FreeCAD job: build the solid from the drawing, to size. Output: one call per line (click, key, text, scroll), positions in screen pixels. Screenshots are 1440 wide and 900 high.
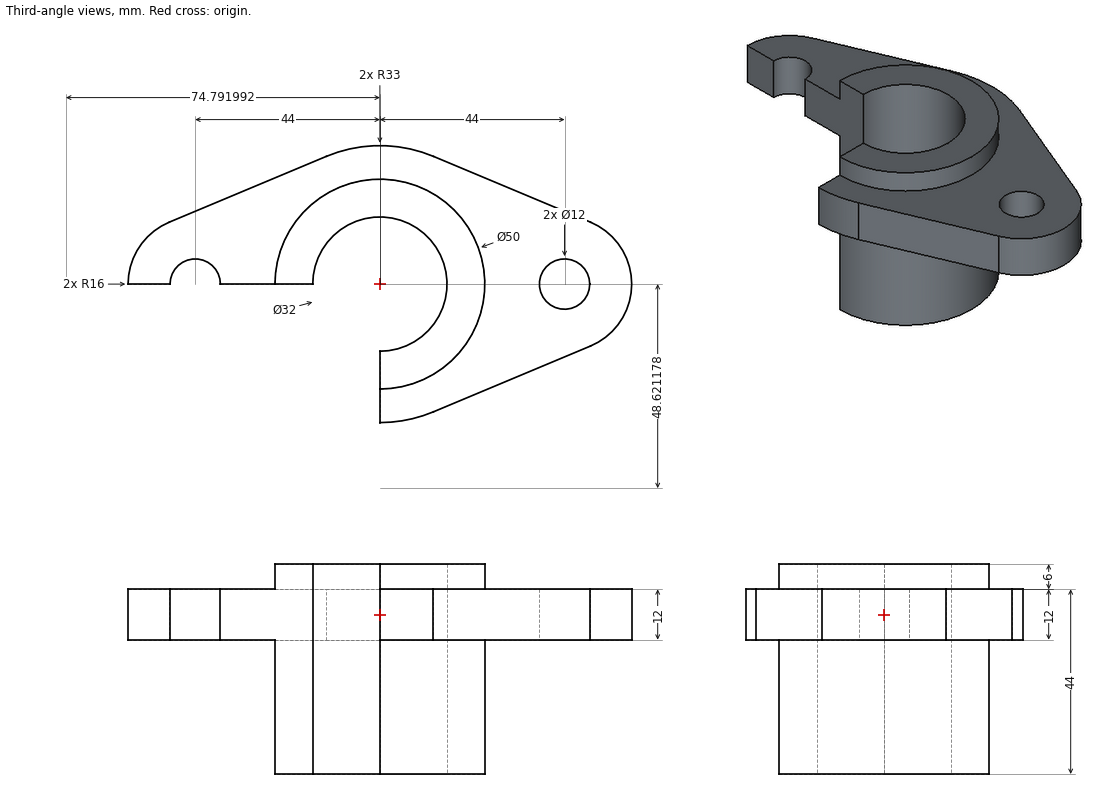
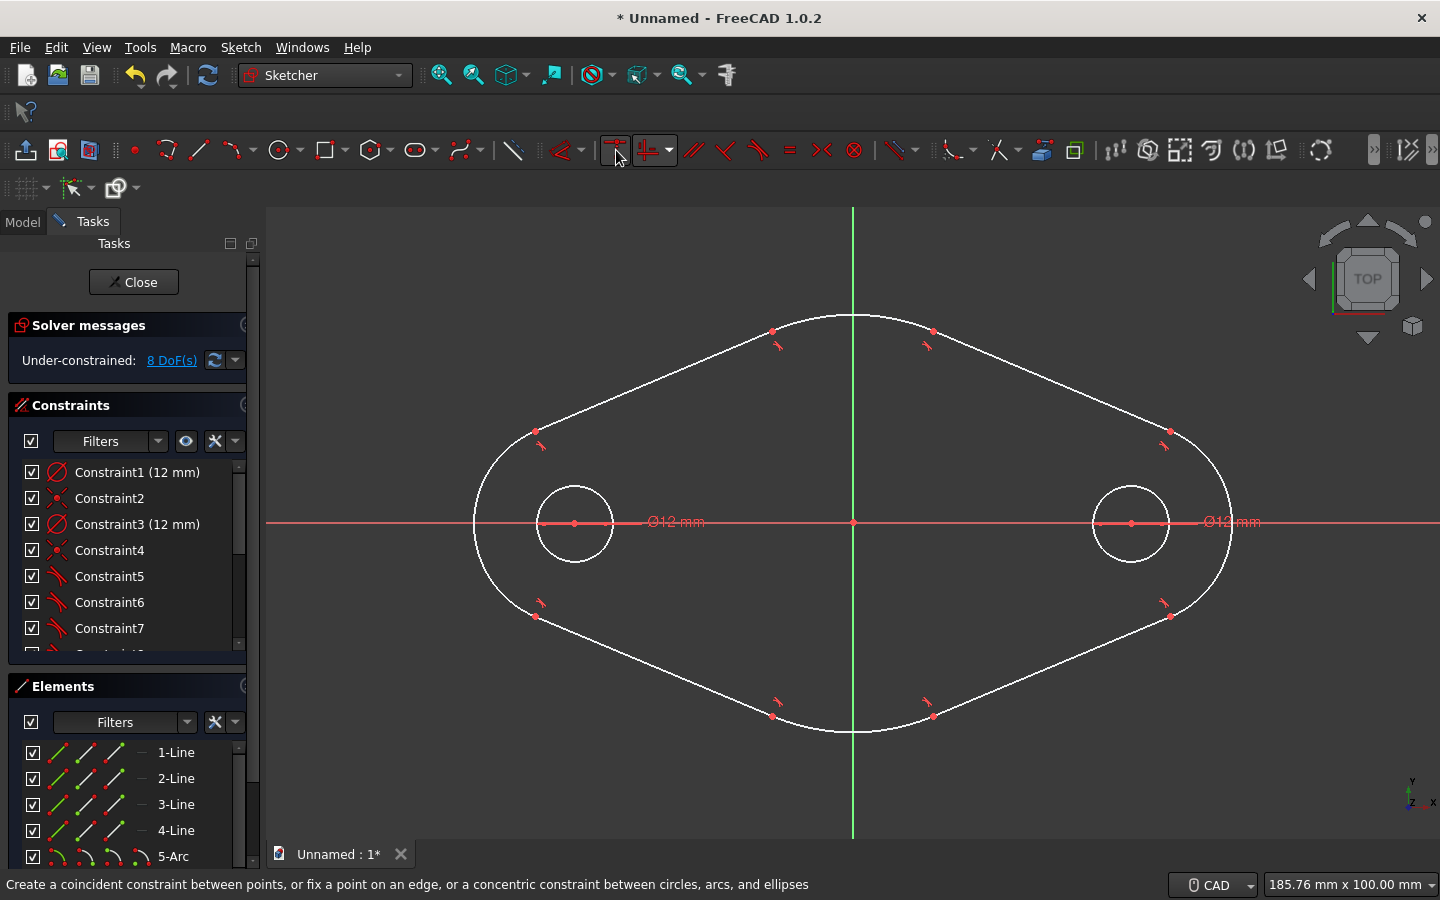
click(886, 317)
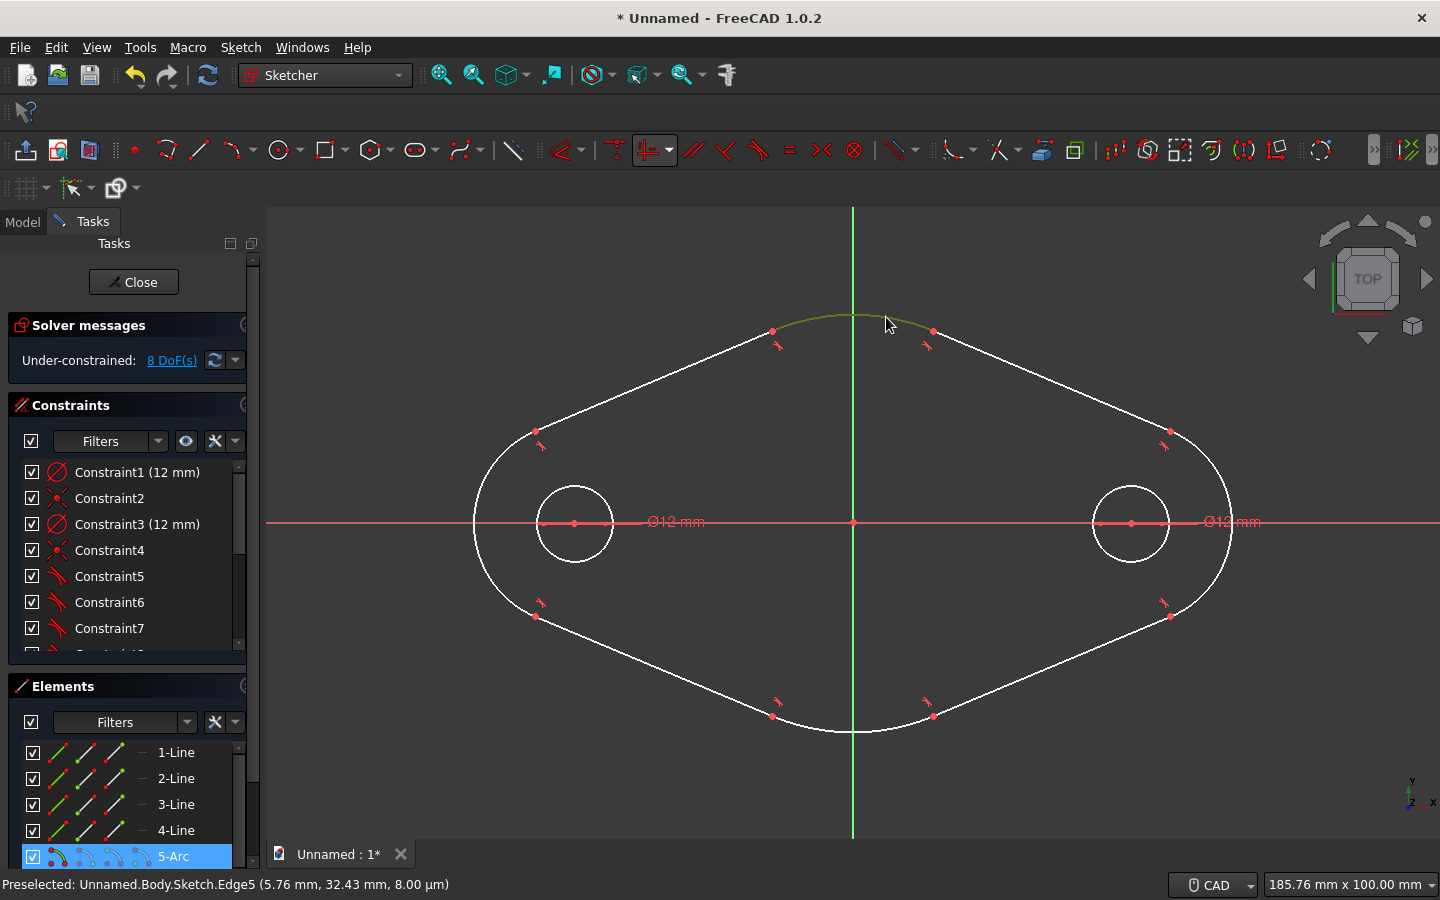
click(820, 730)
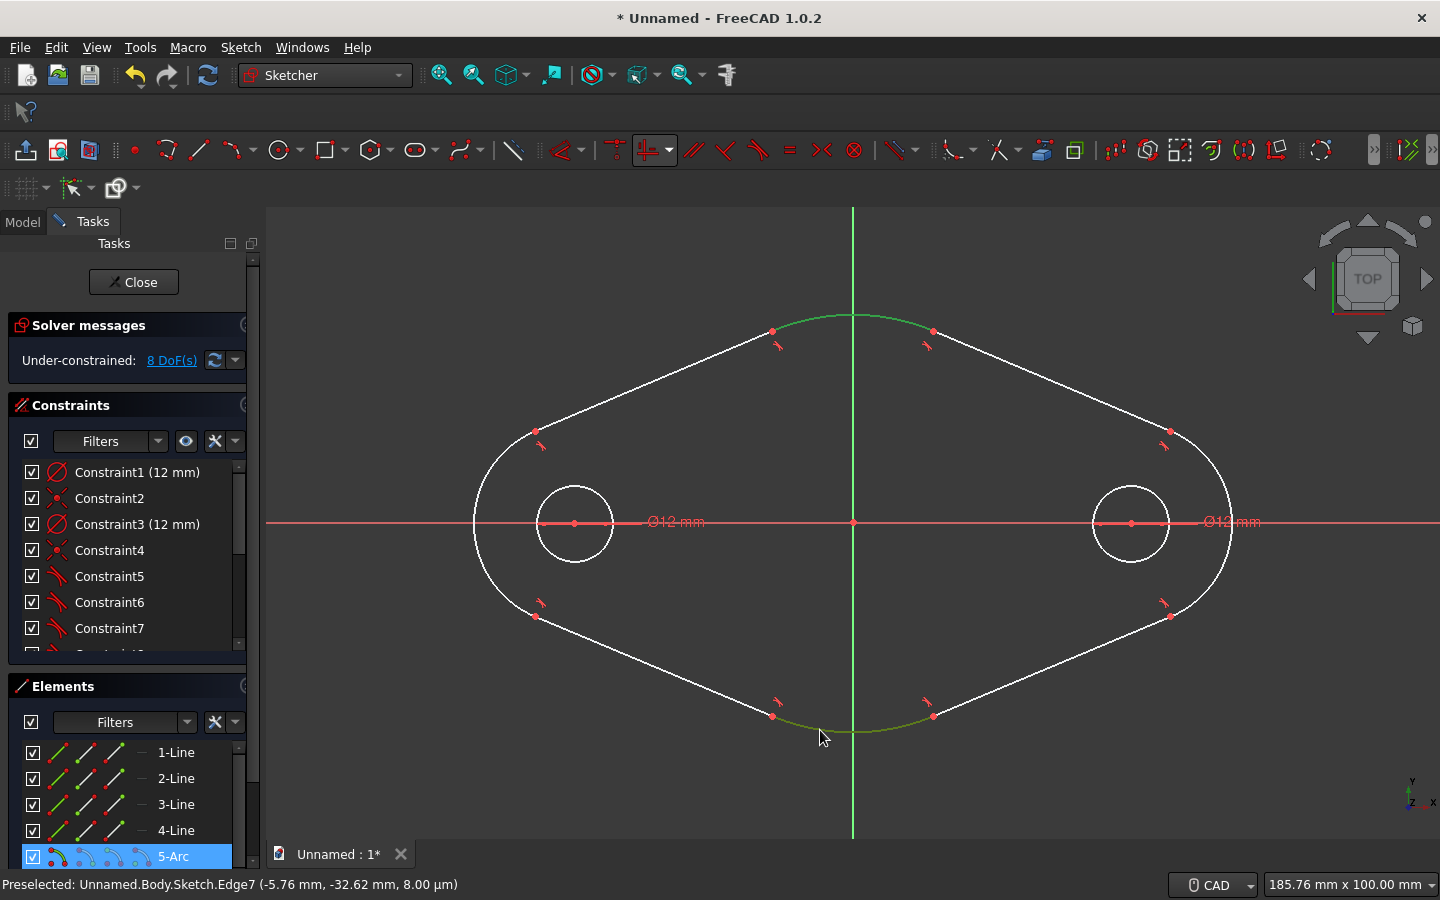
click(790, 150)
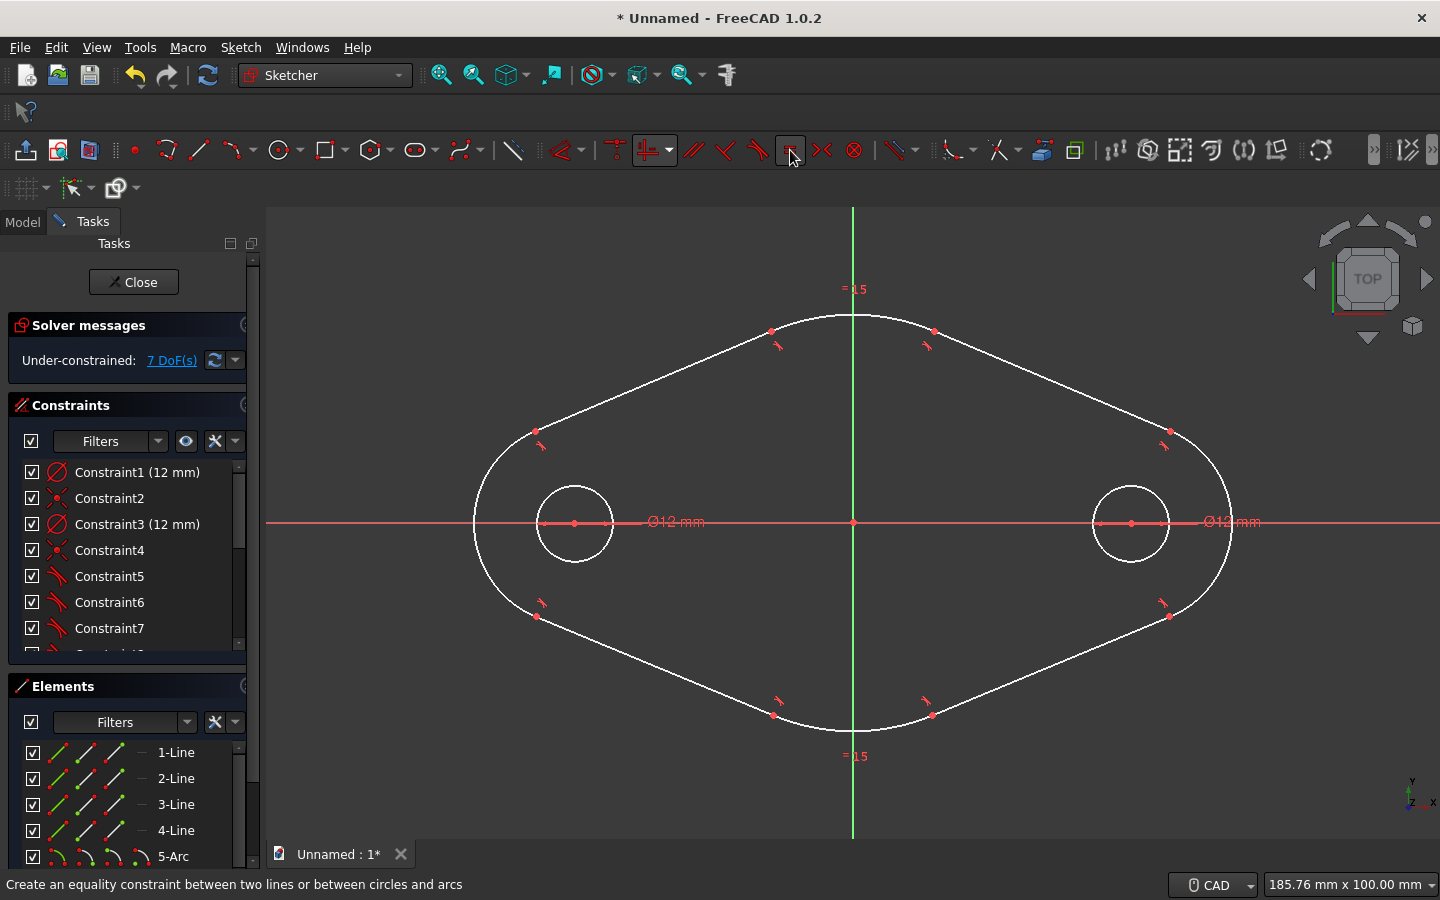
click(485, 479)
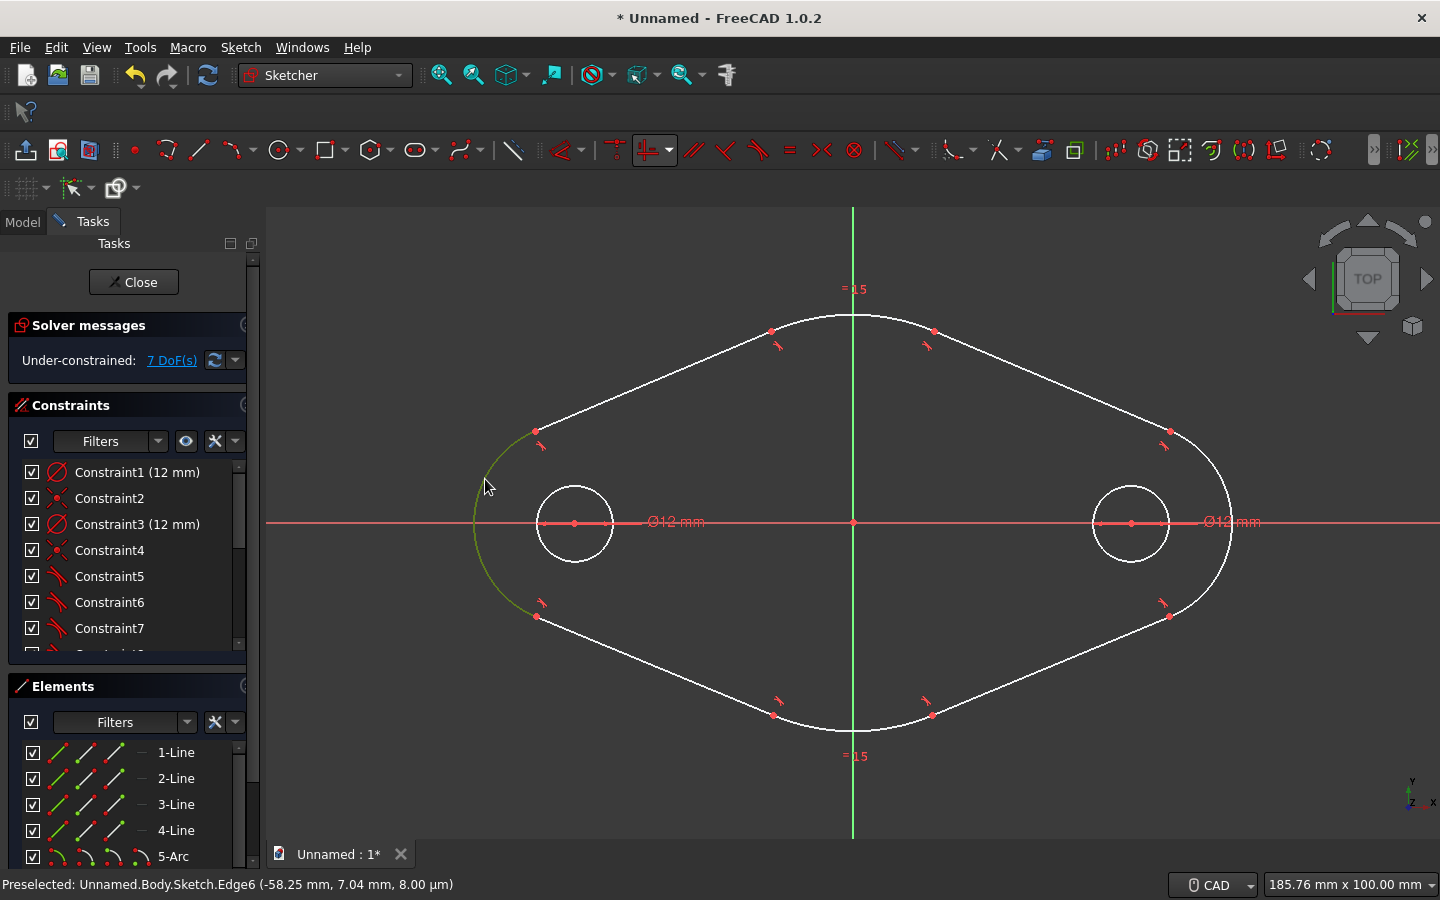
click(1221, 570)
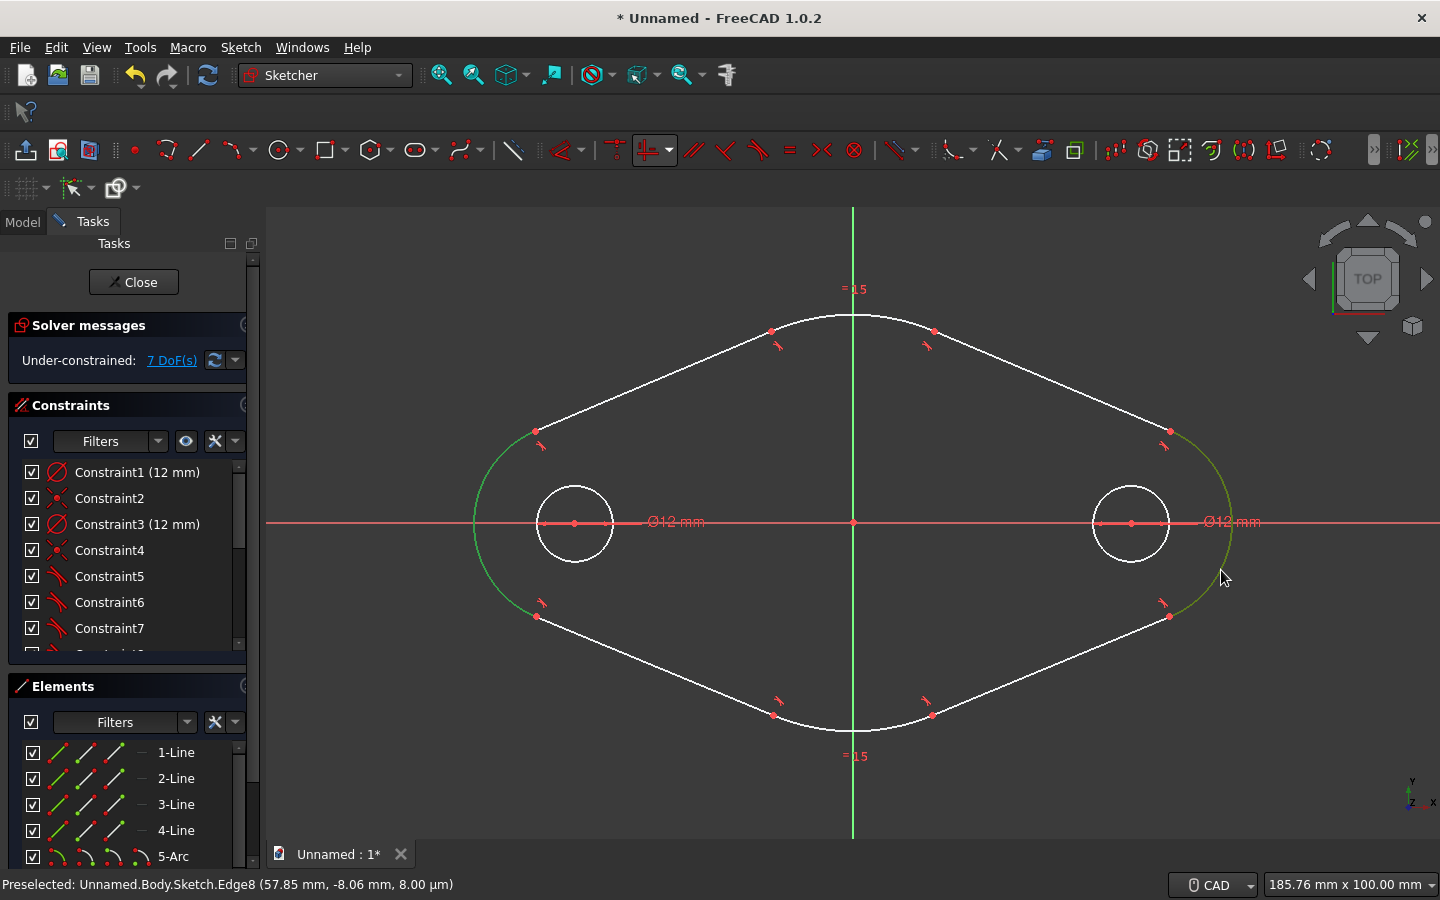
click(790, 150)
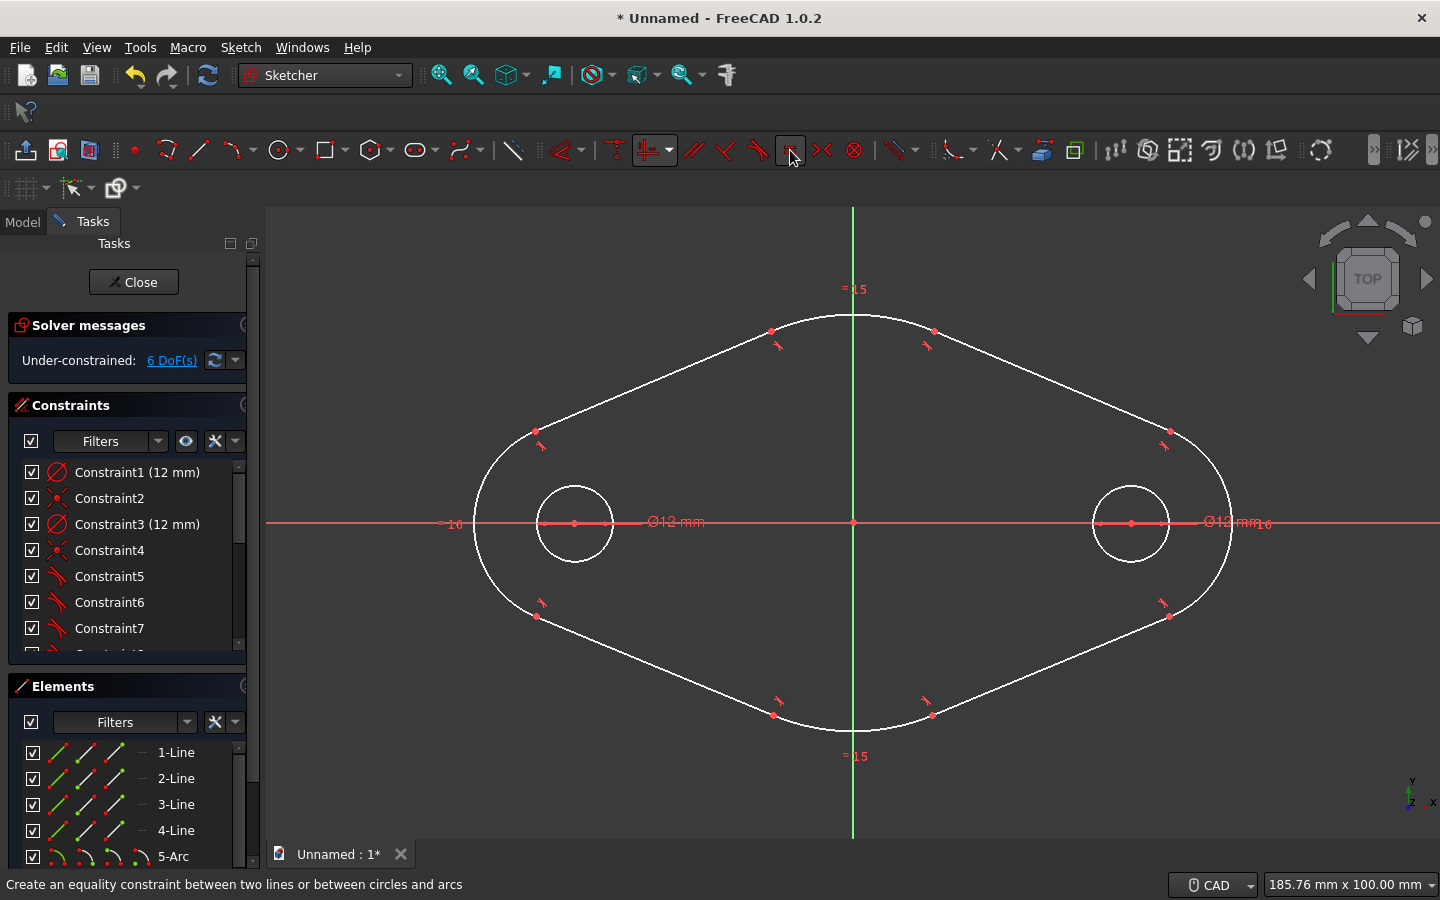
click(575, 524)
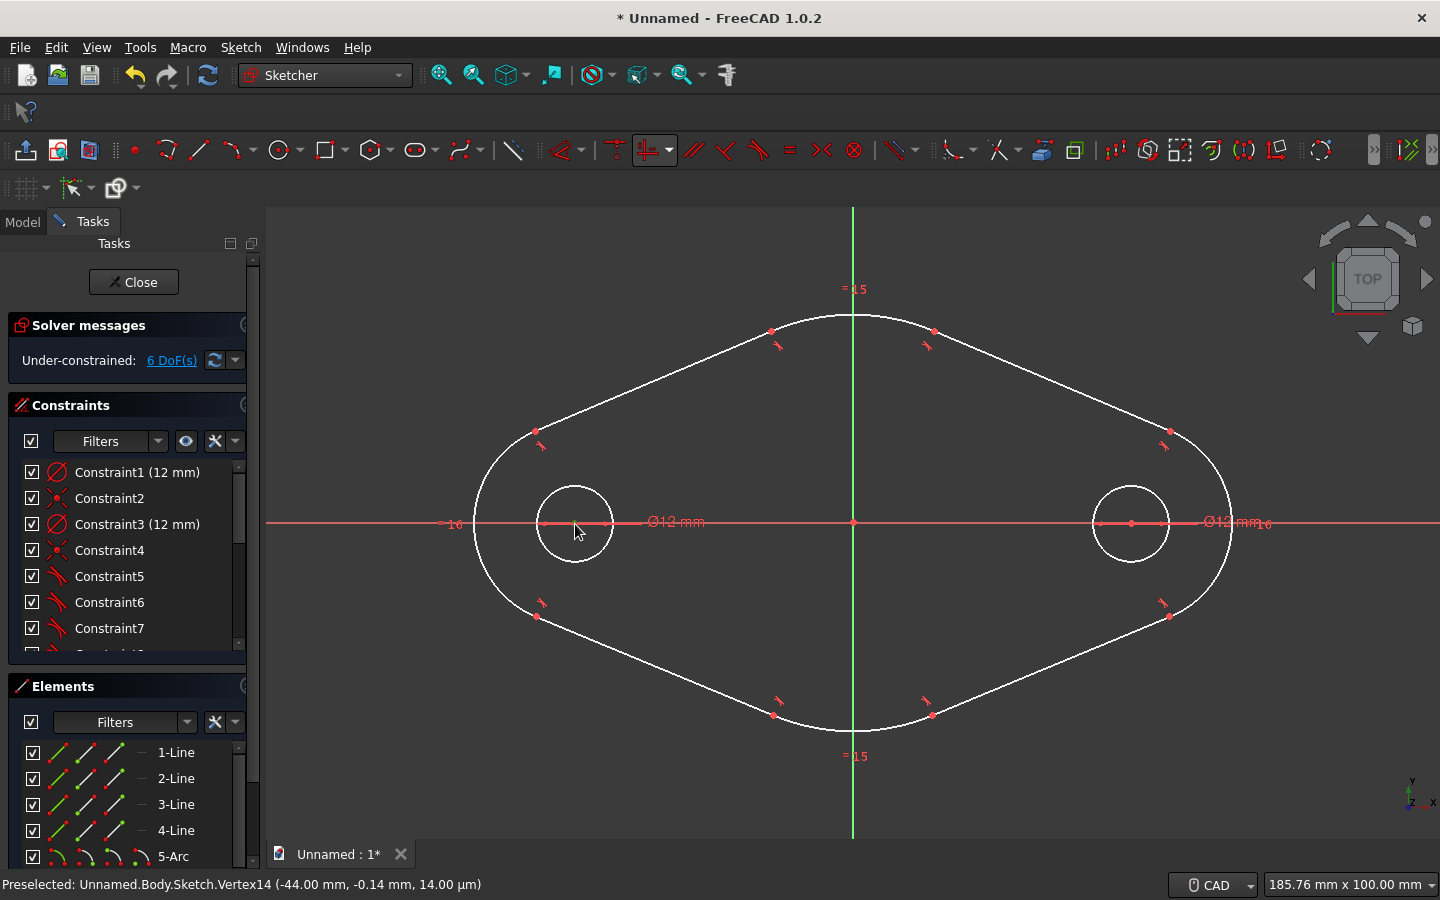
click(364, 523)